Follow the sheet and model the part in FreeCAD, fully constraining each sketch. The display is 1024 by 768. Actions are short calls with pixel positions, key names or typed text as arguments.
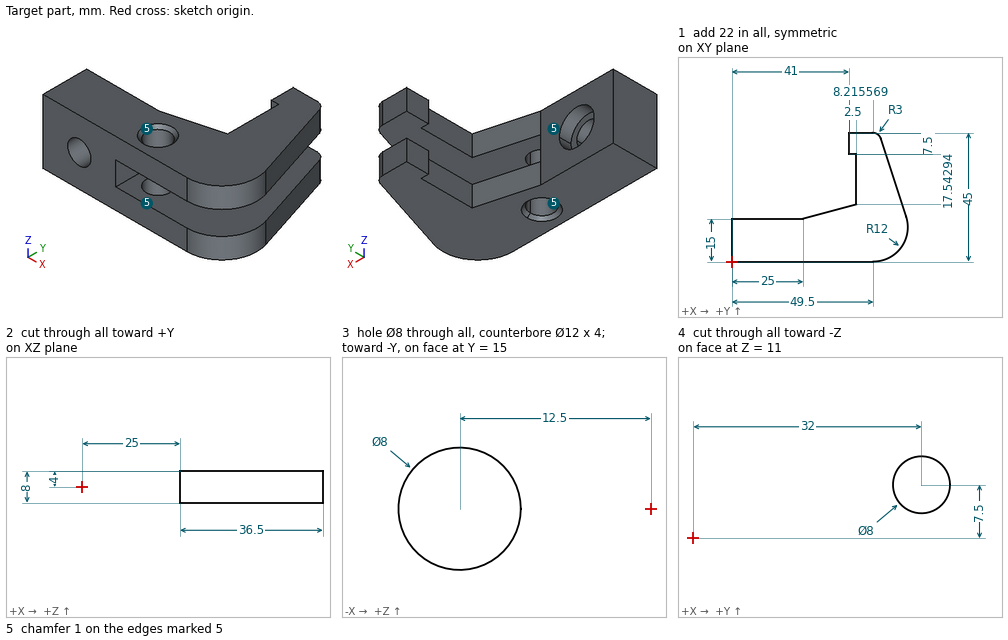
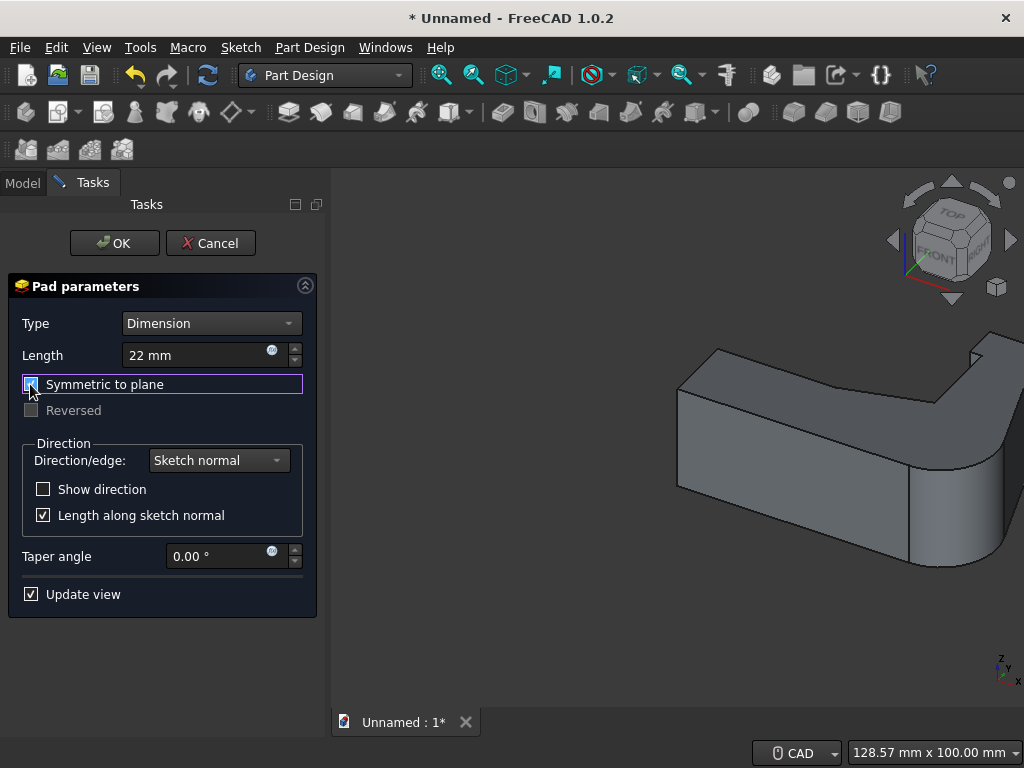
click(115, 243)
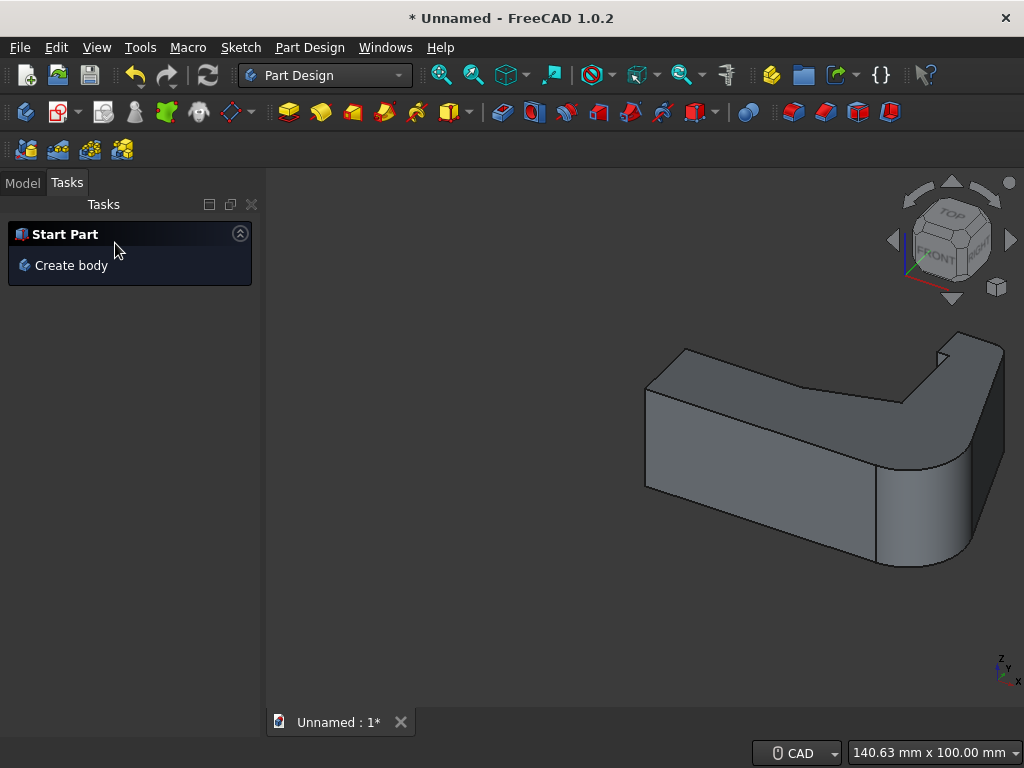
key(v)
key(f)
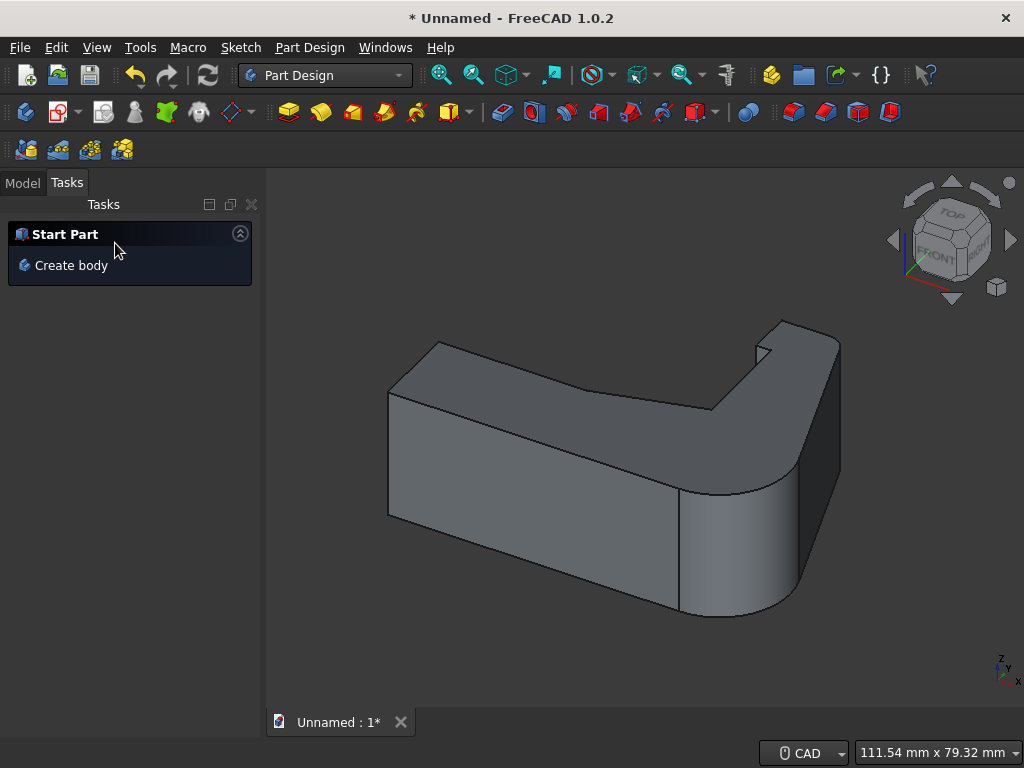
click(58, 112)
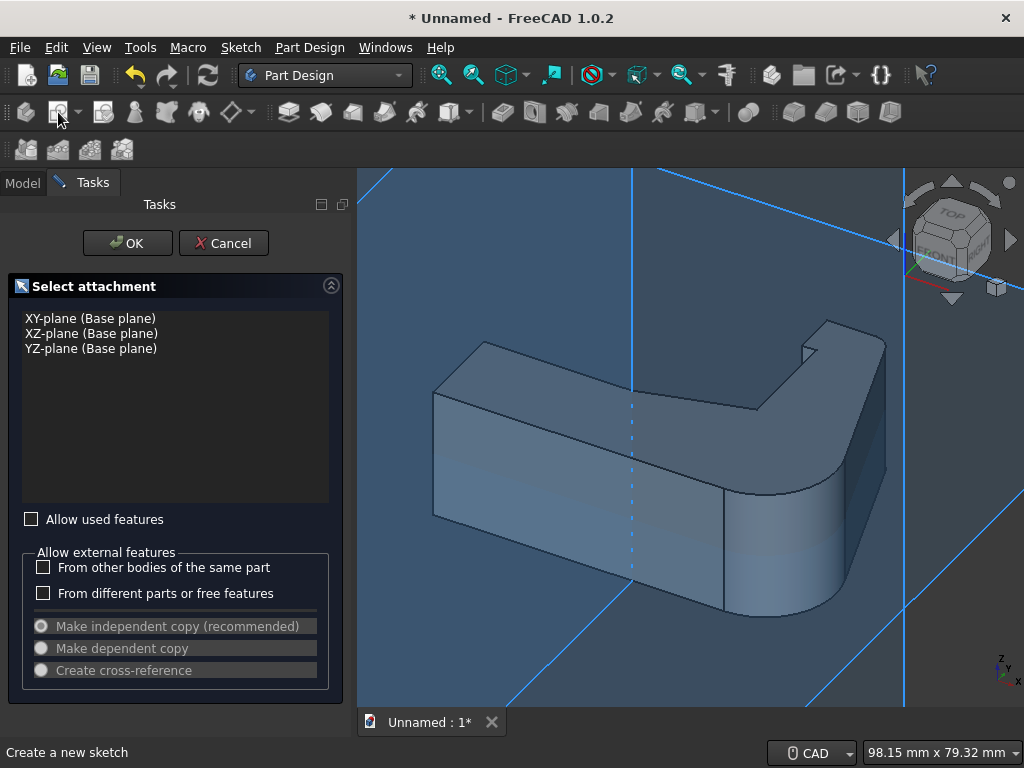
click(82, 334)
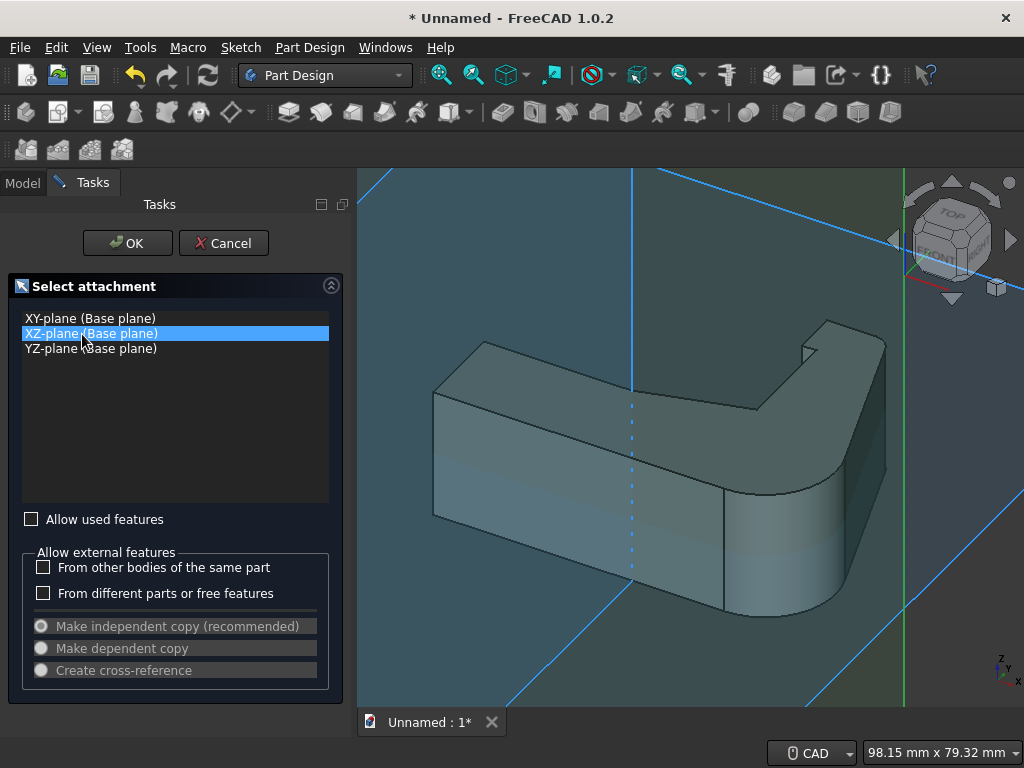
click(128, 243)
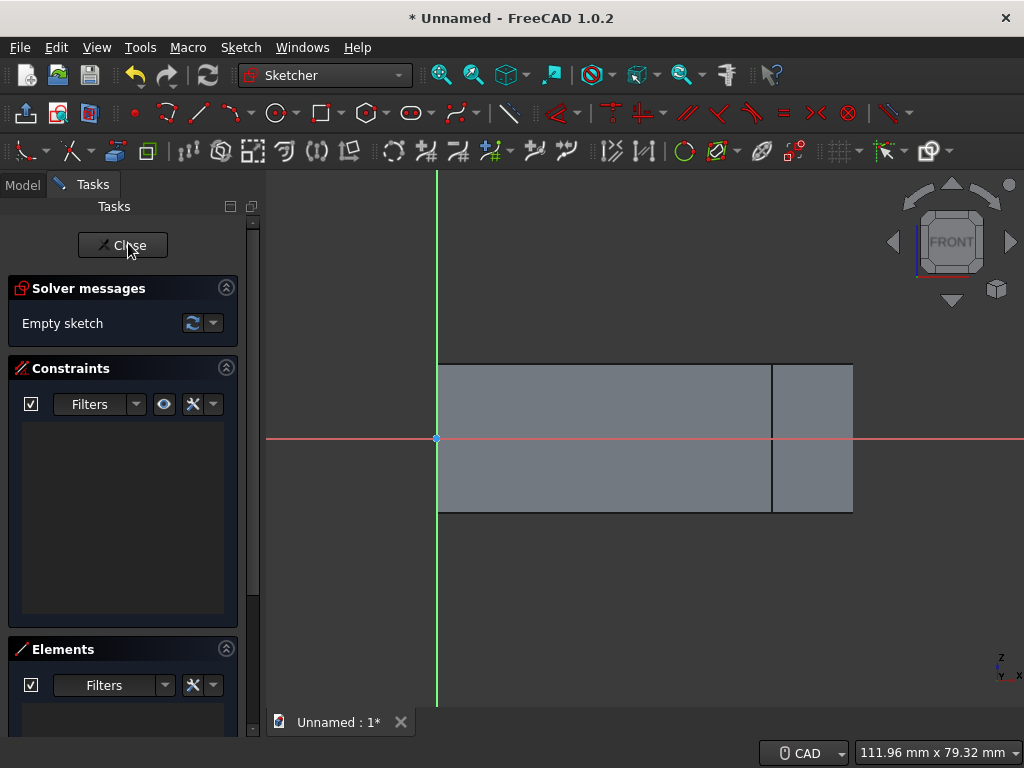
scroll(294, 439, down, 1)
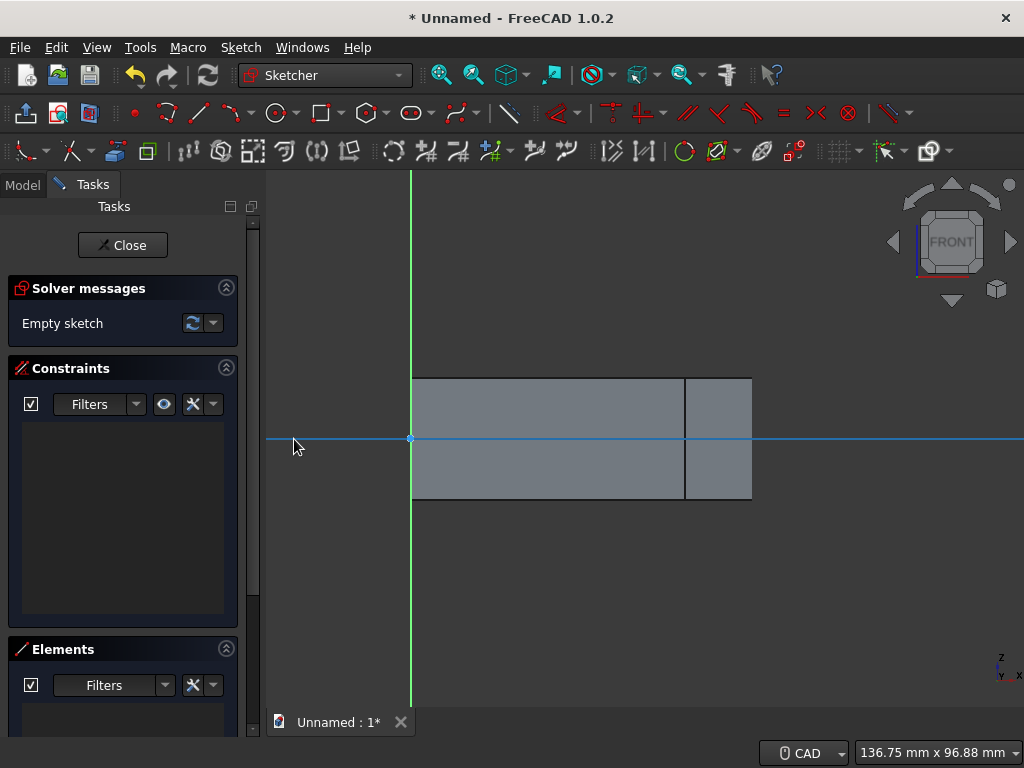
key(g)
key(r)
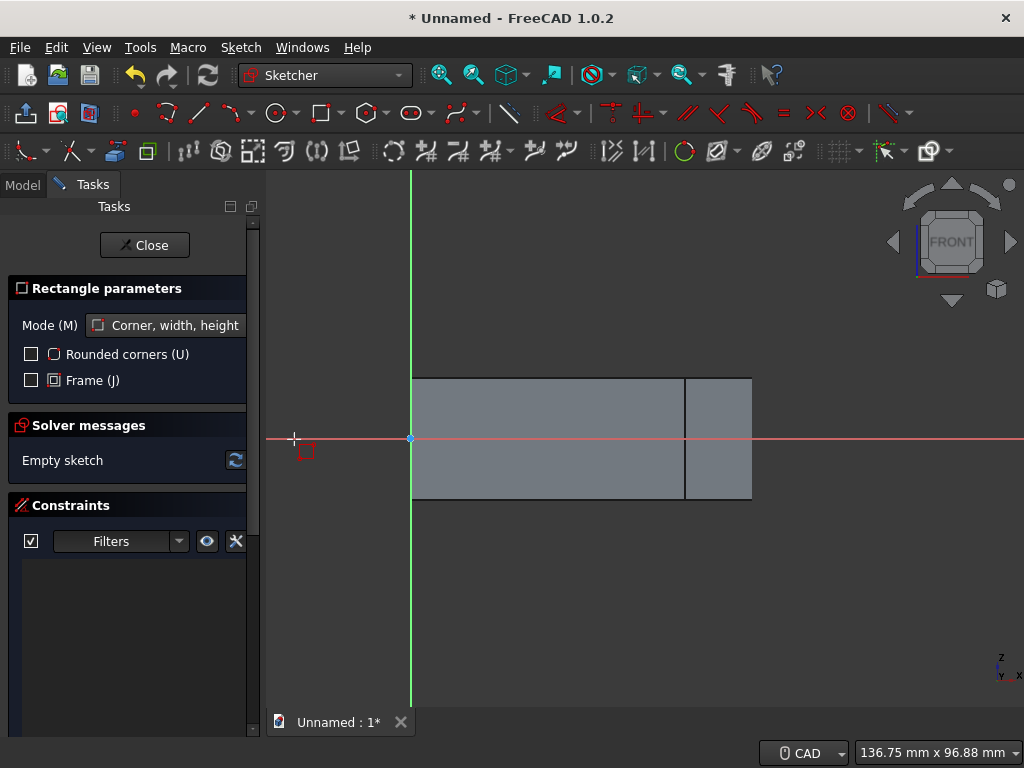
click(550, 417)
click(752, 461)
key(Escape)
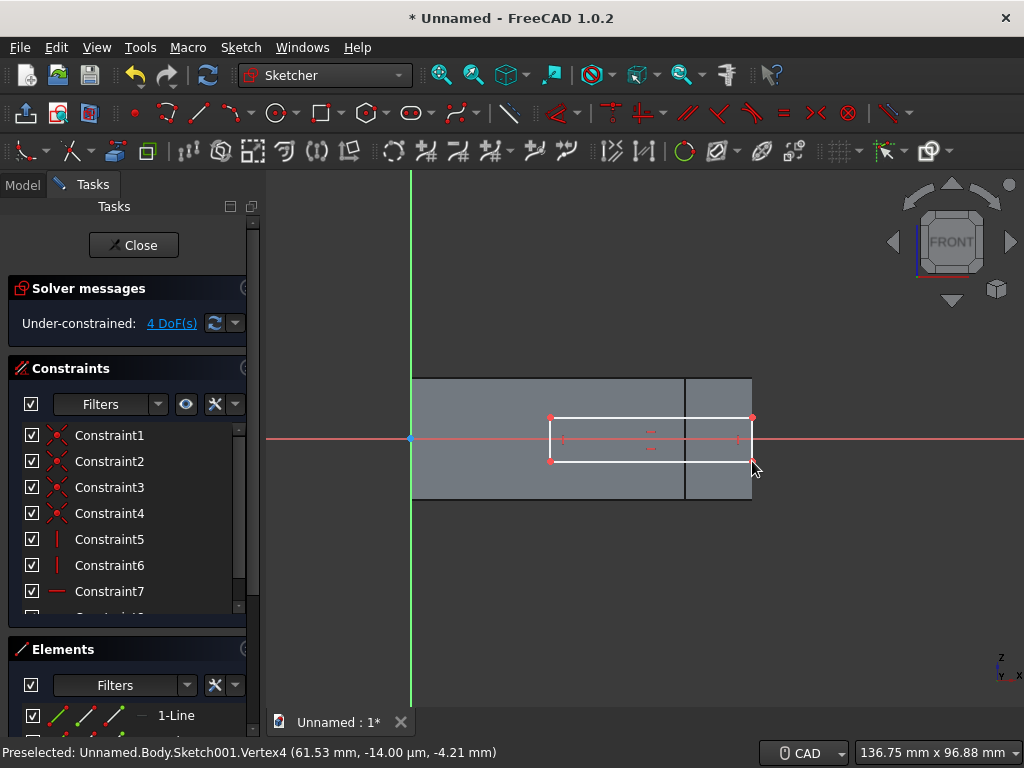
scroll(550, 449, up, 2)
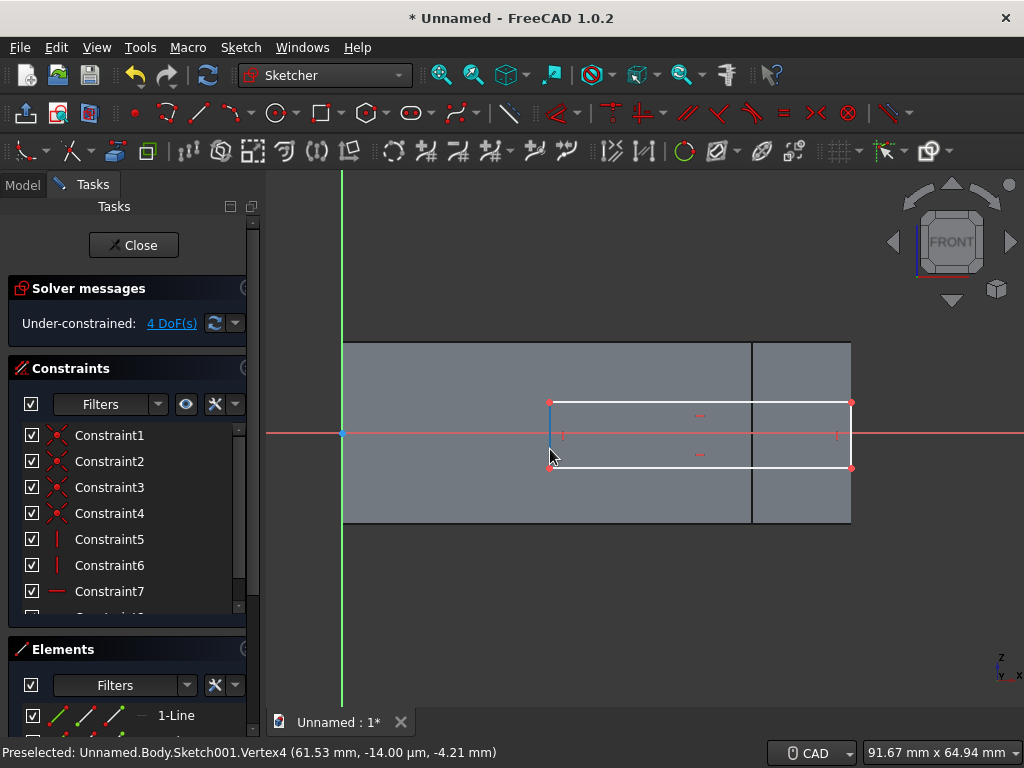
click(550, 448)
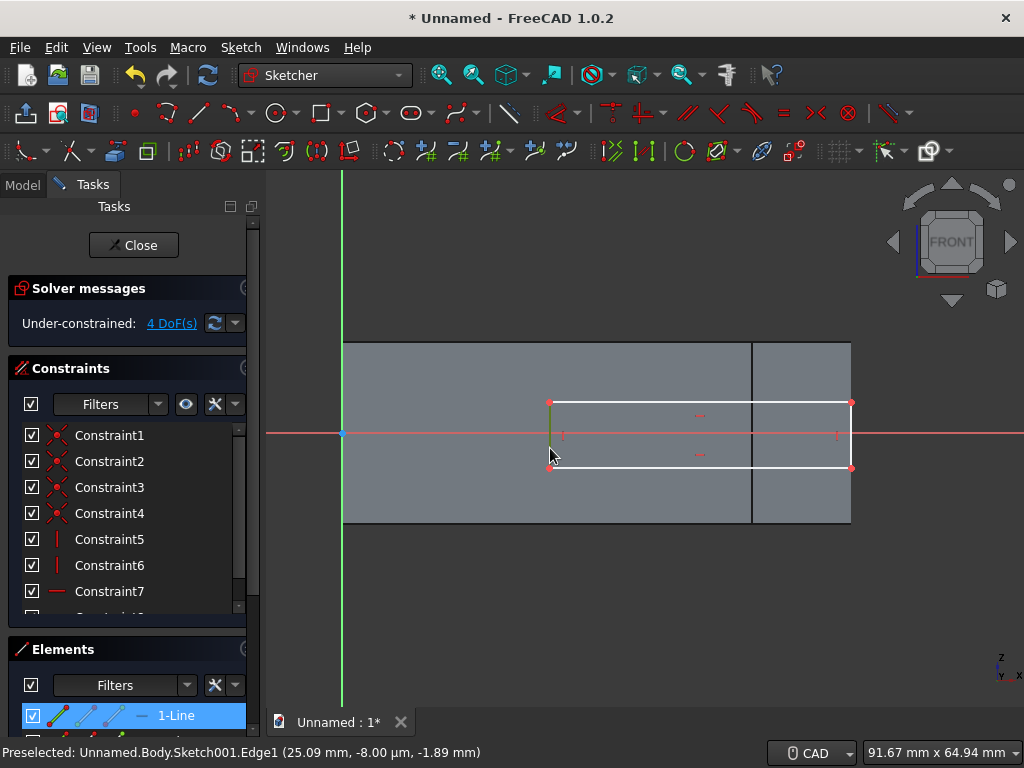
key(i)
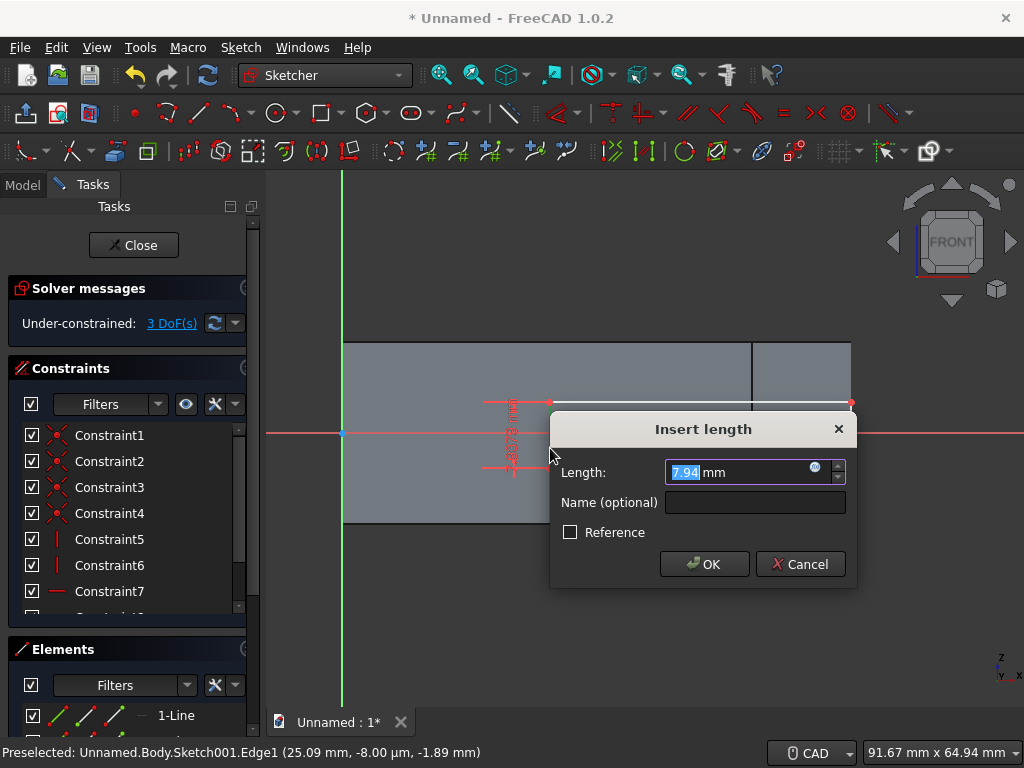
text(8)
key(Return)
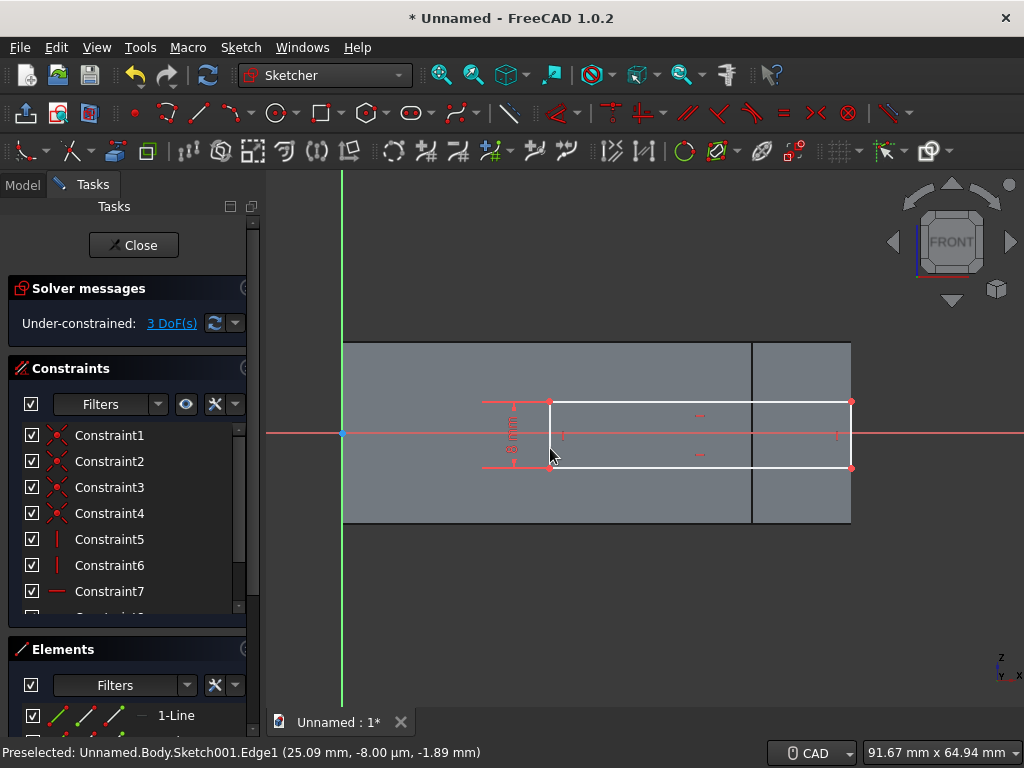
click(550, 402)